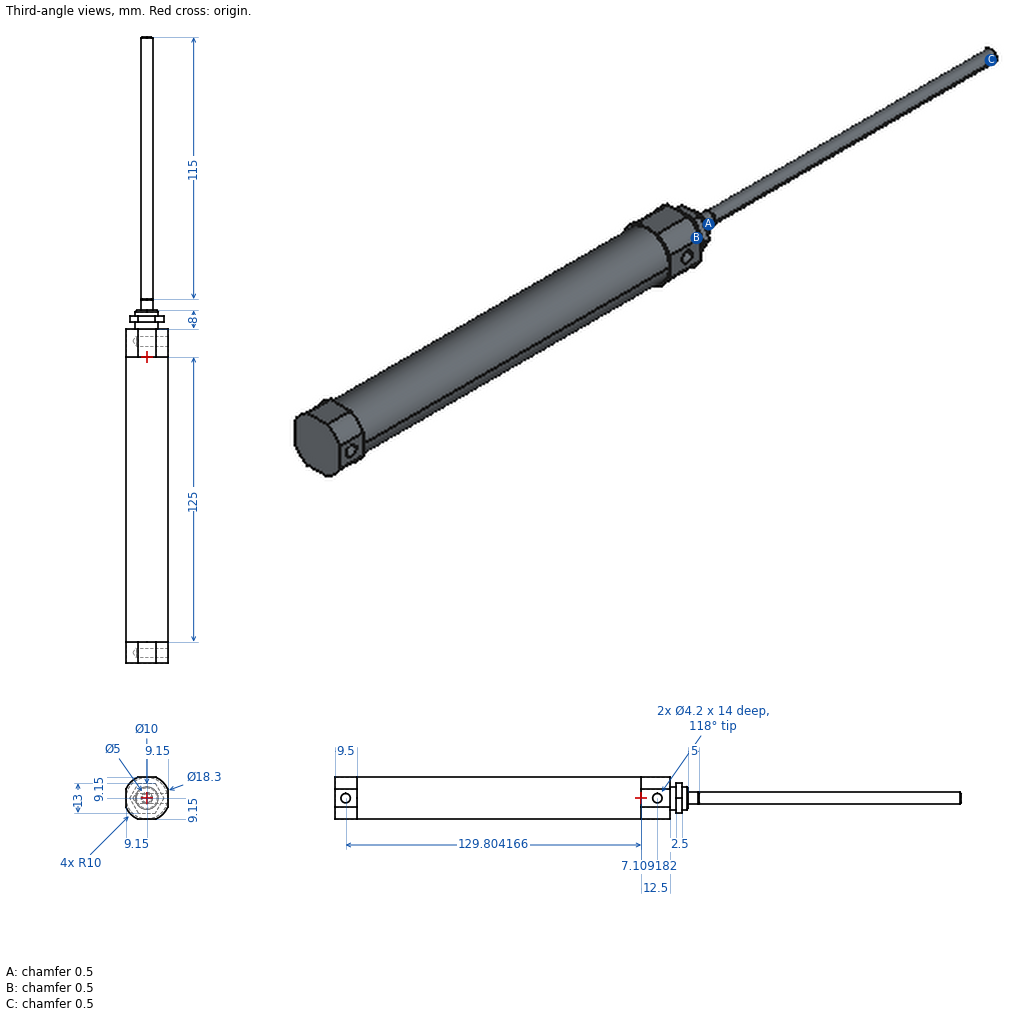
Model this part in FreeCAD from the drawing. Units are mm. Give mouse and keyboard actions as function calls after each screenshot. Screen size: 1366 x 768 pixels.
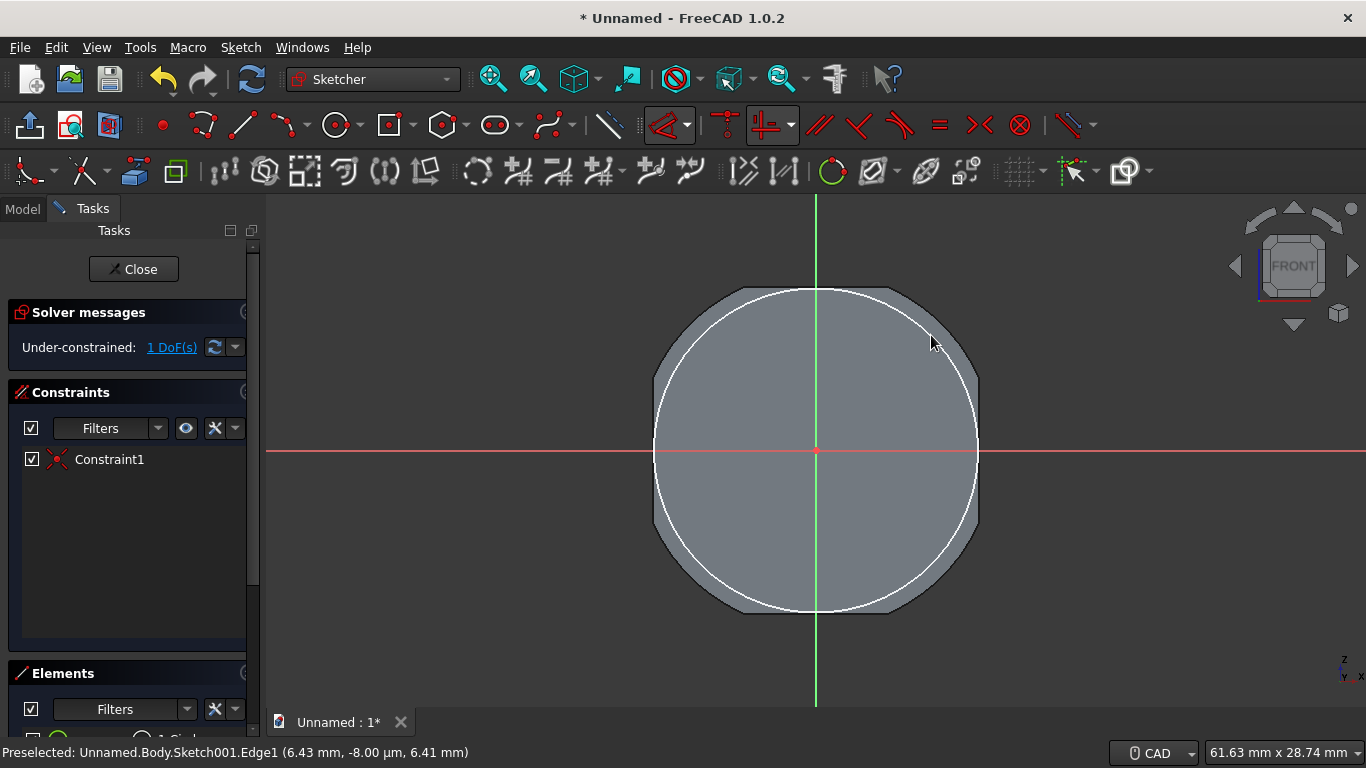
key(d)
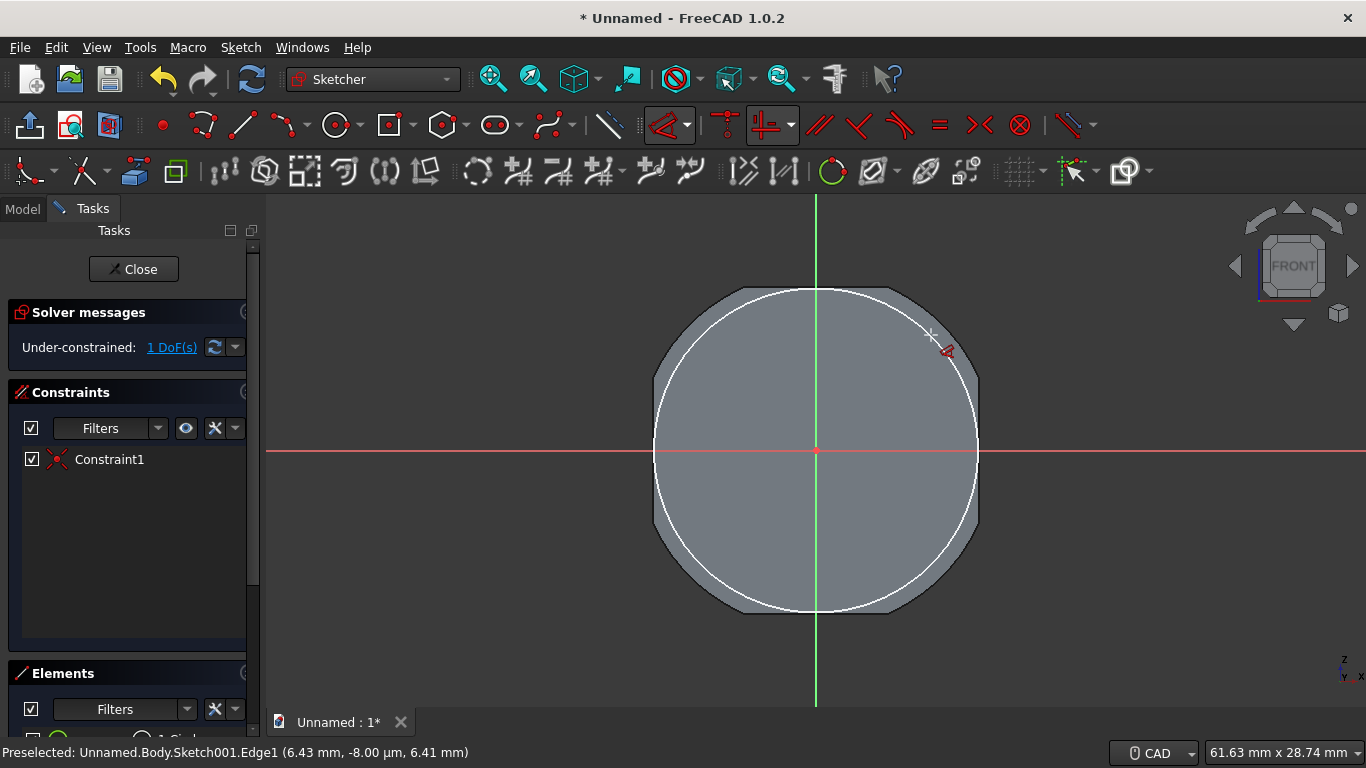
click(930, 335)
click(952, 312)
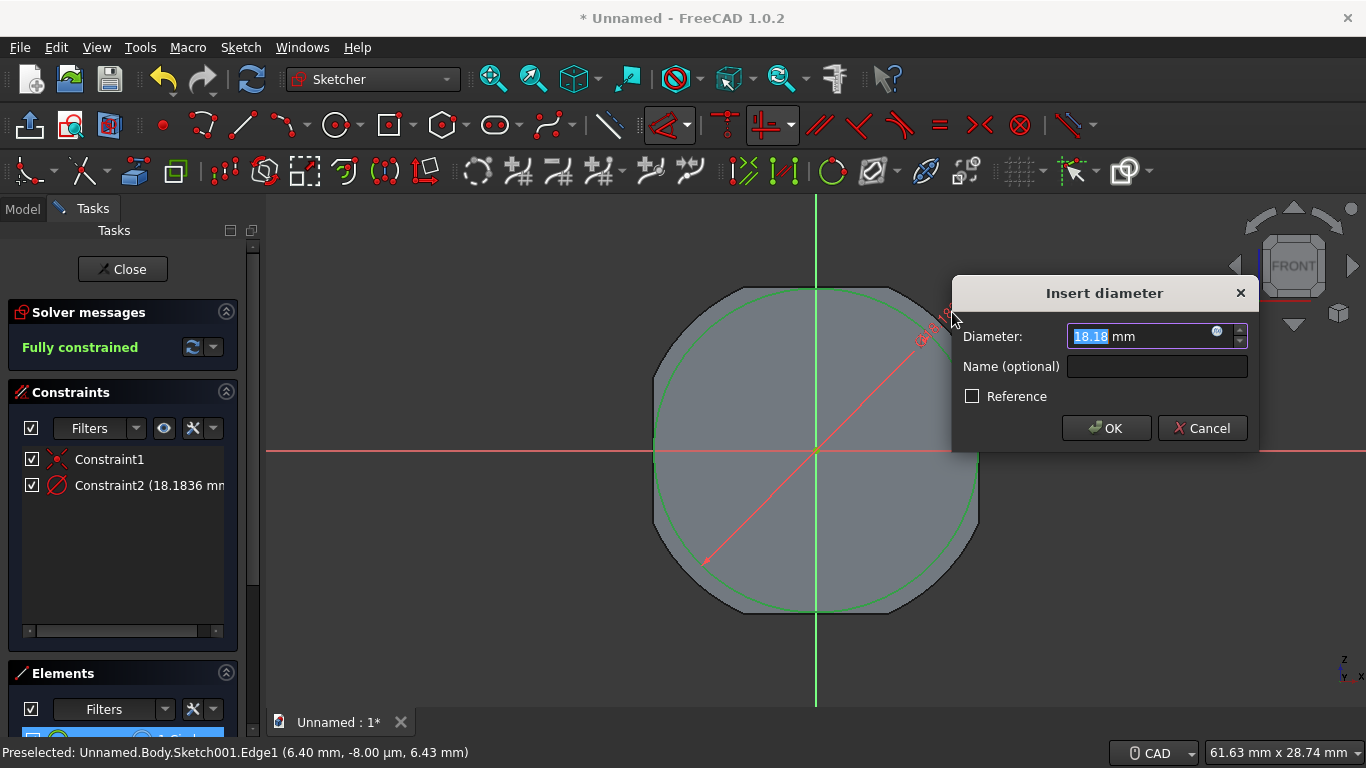
text(18.3)
key(Return)
key(Escape)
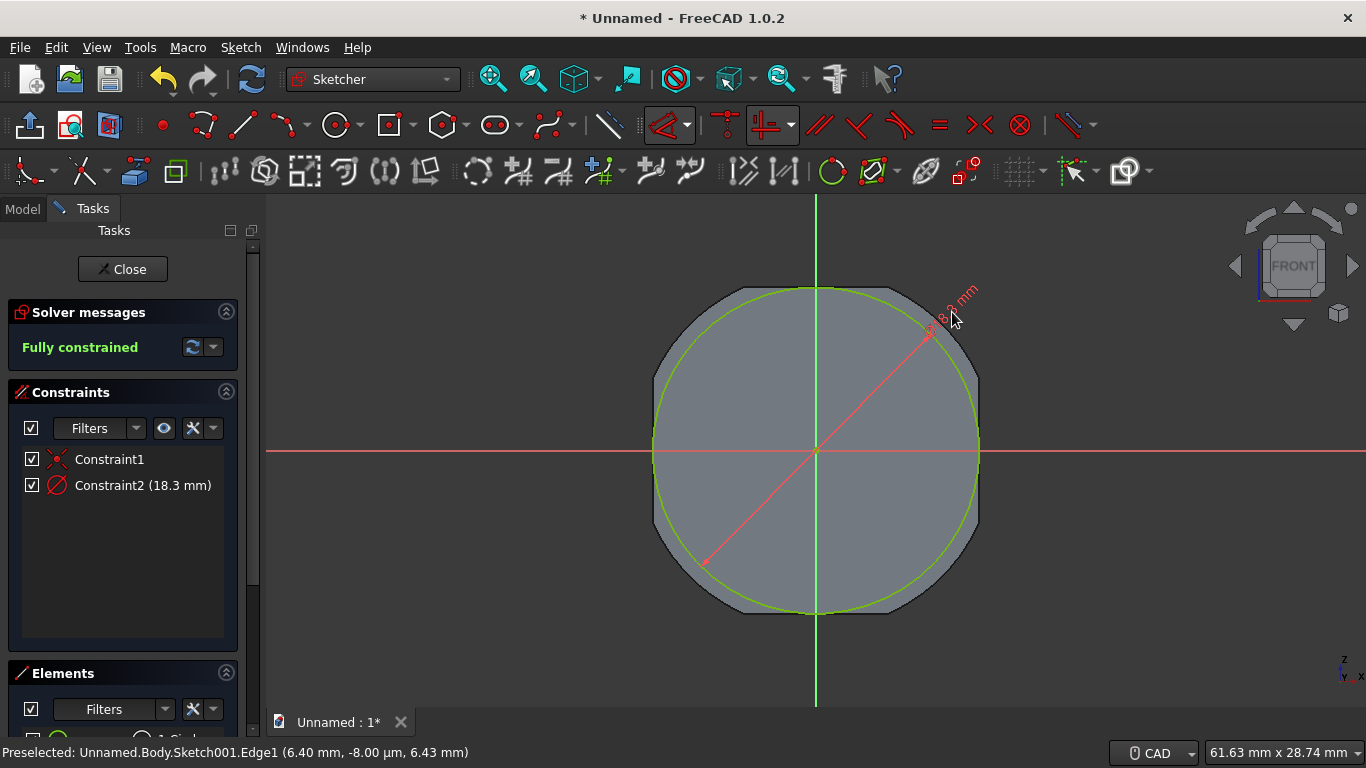
click(123, 269)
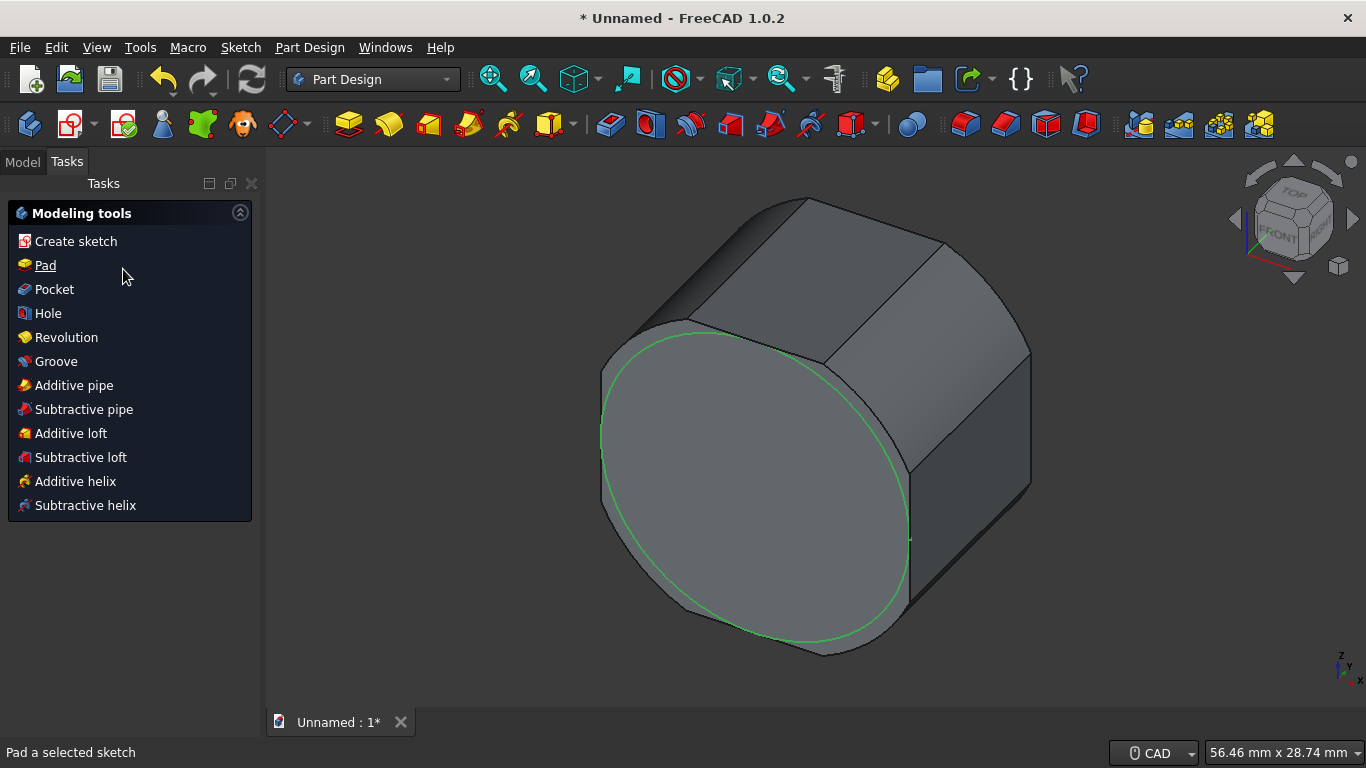
click(350, 124)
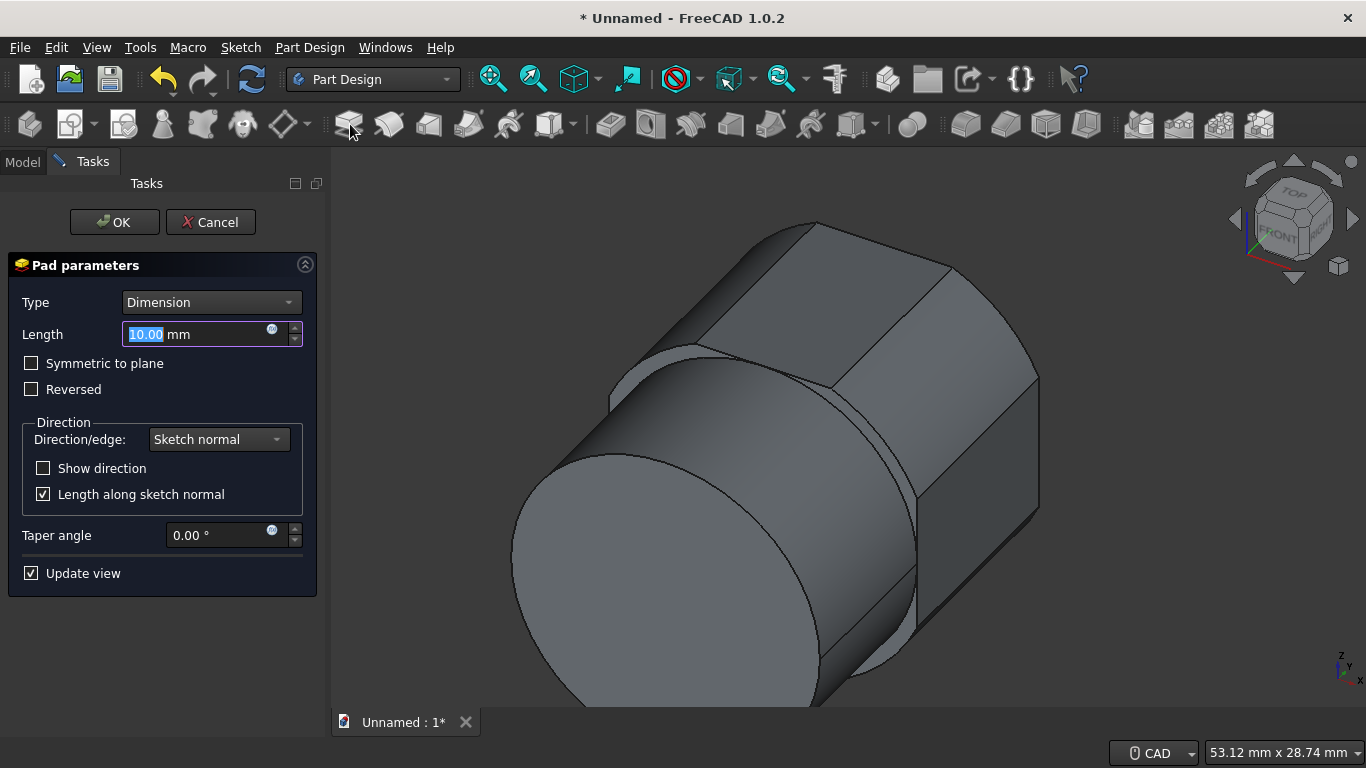
text(125)
key(Tab)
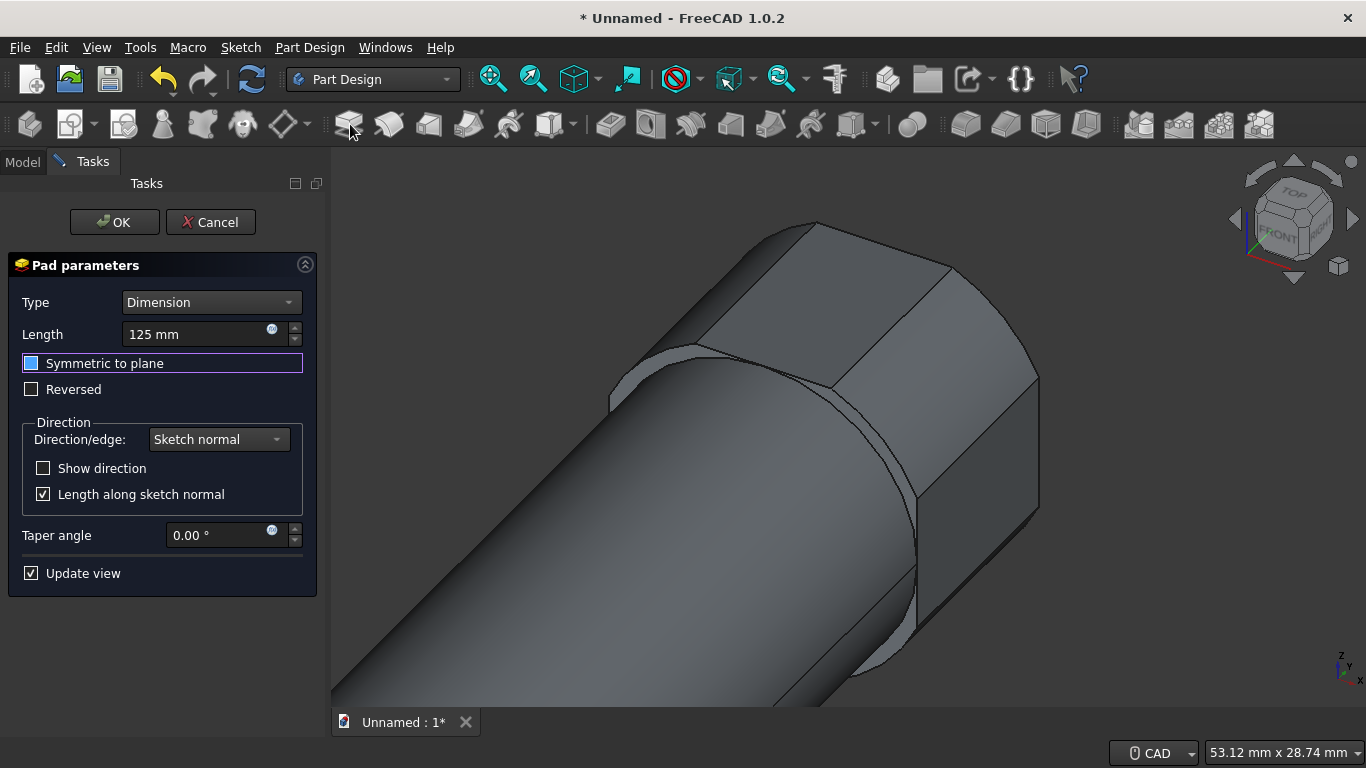
click(115, 222)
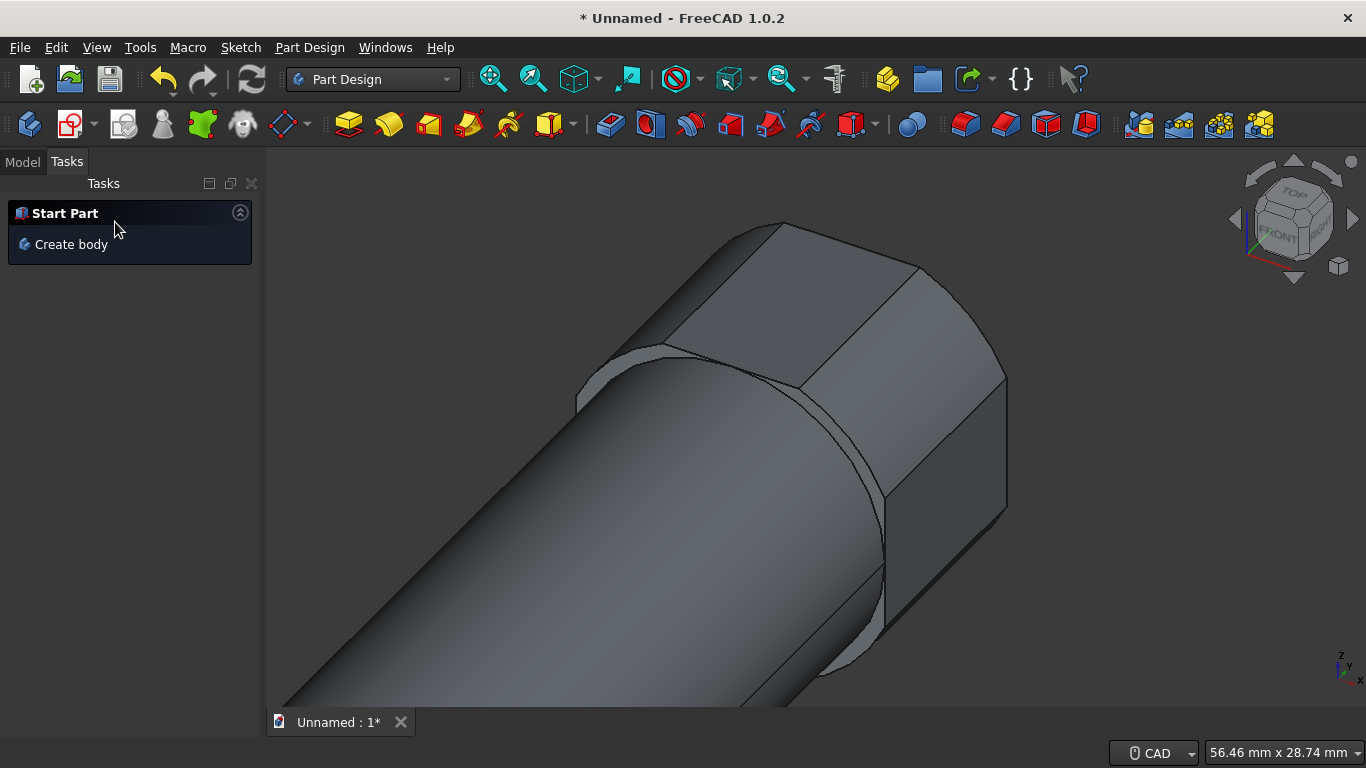
key(v)
key(f)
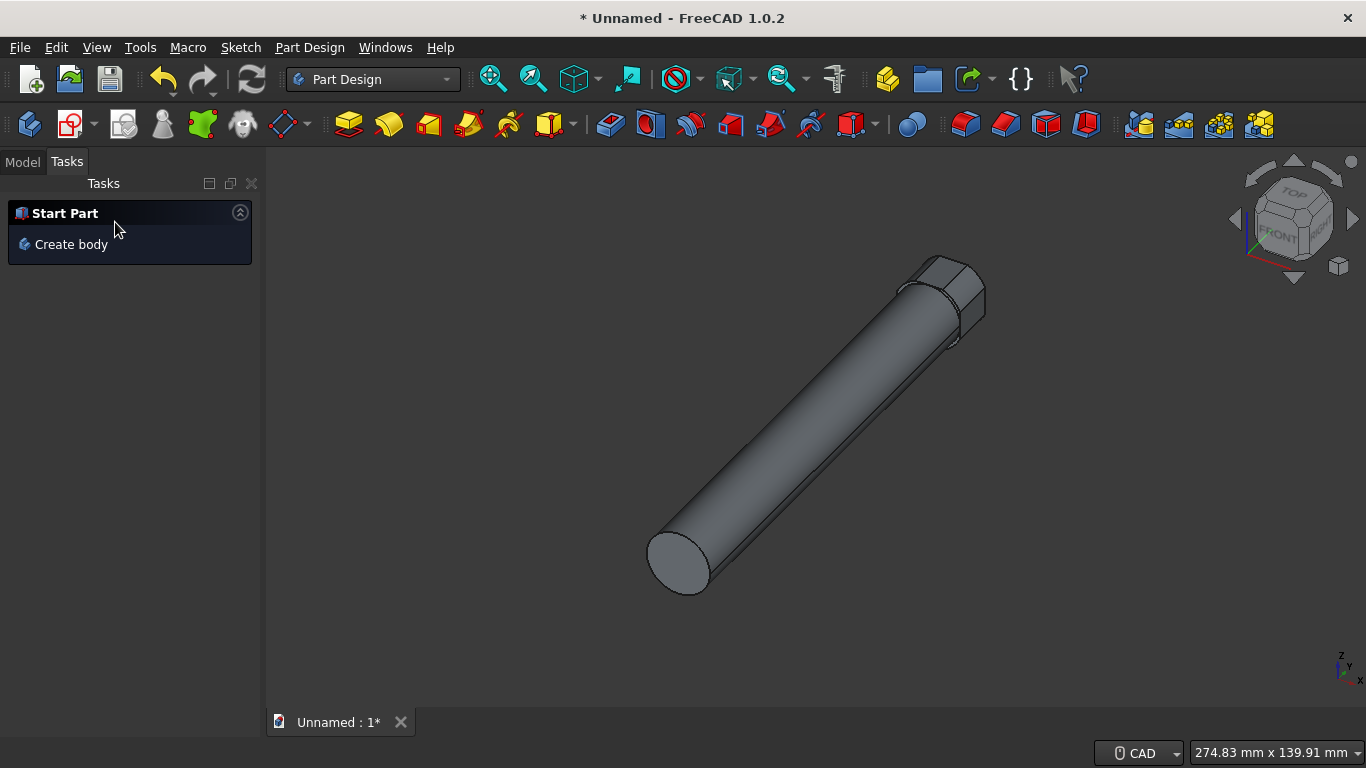
click(23, 161)